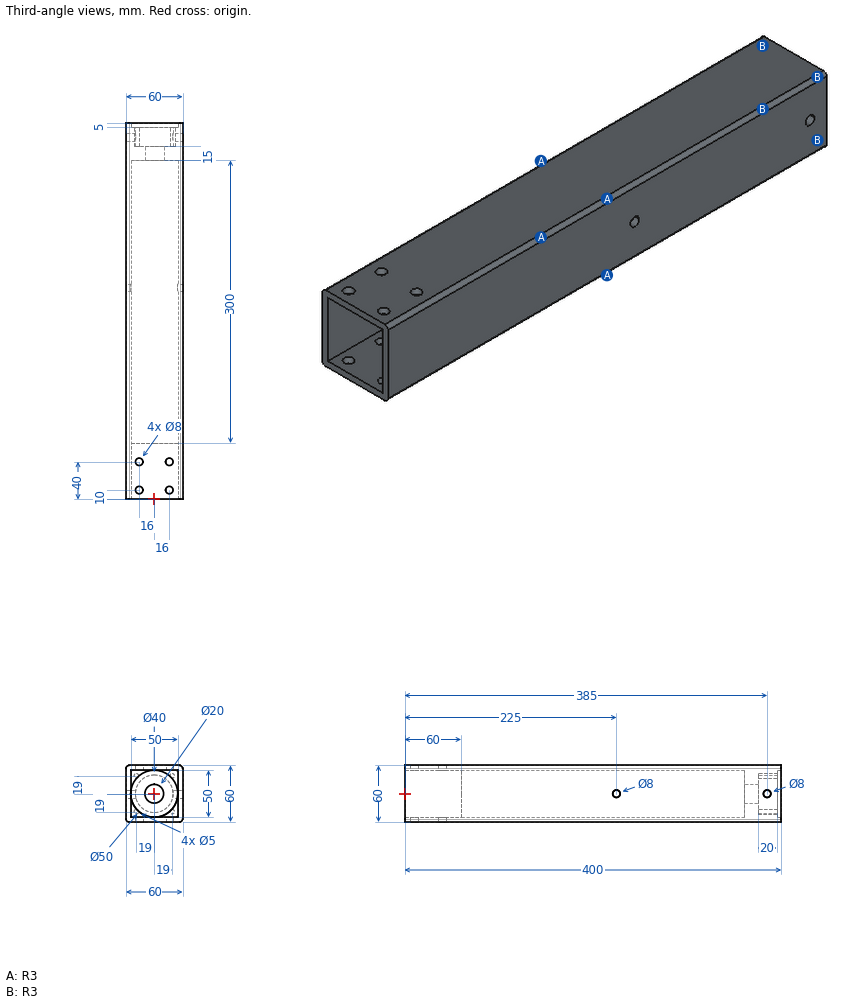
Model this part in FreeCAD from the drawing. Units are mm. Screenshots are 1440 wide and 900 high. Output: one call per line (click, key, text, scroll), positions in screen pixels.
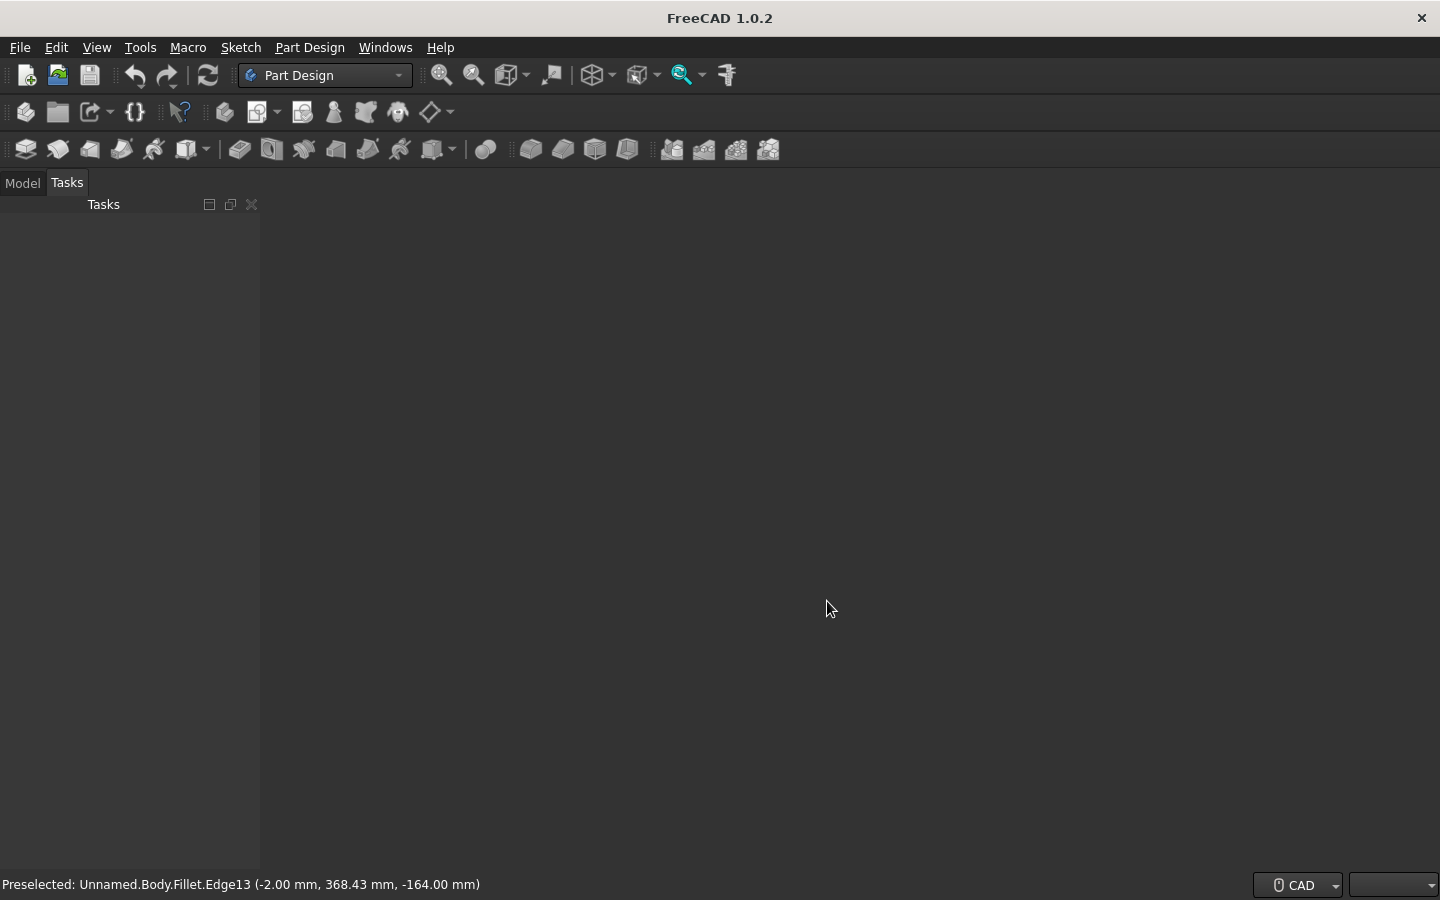
click(26, 76)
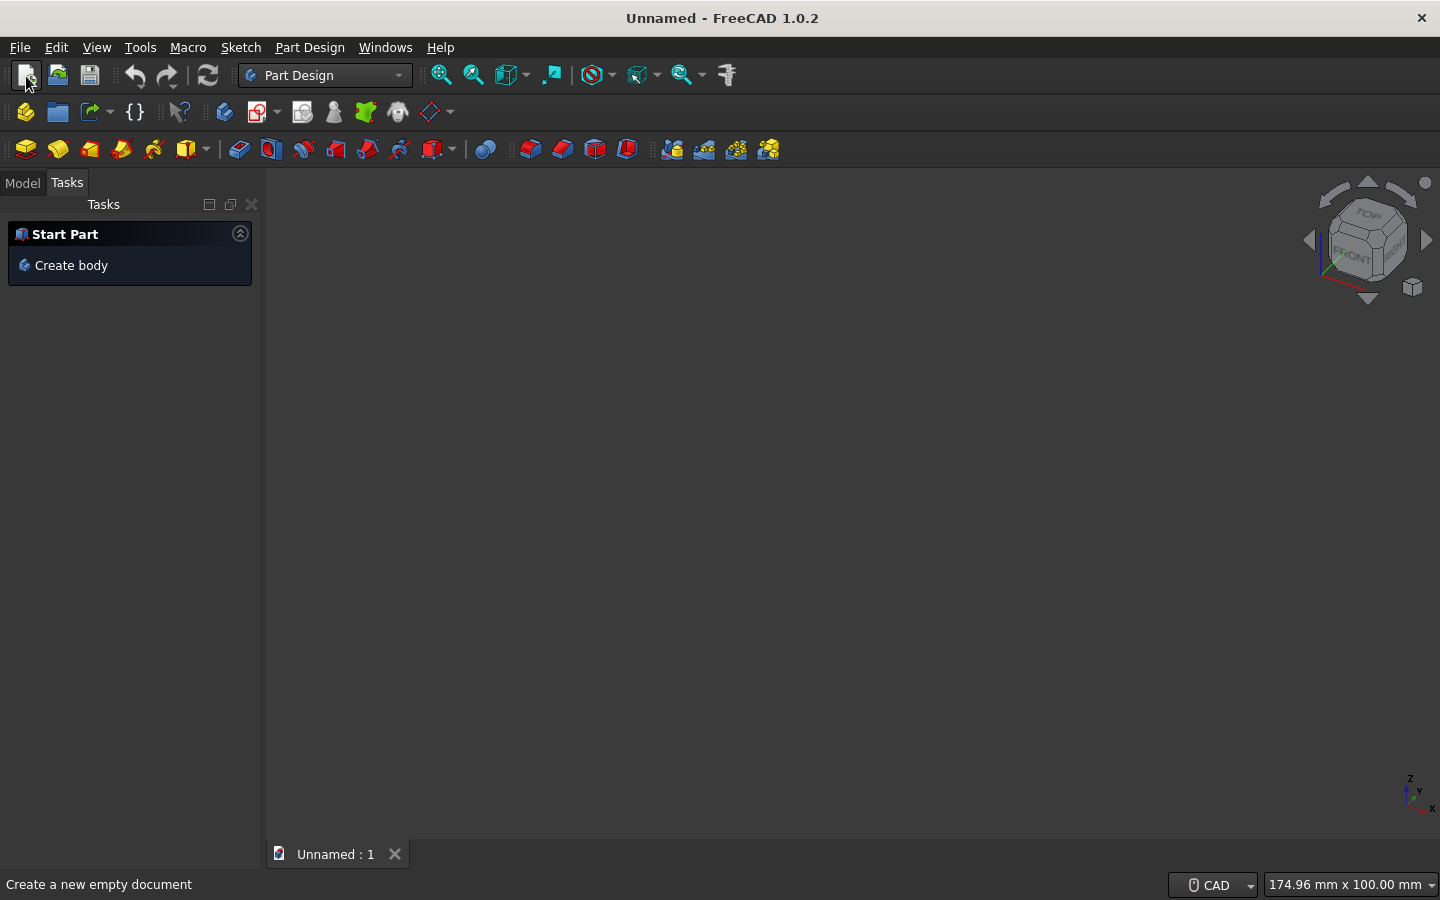
click(258, 112)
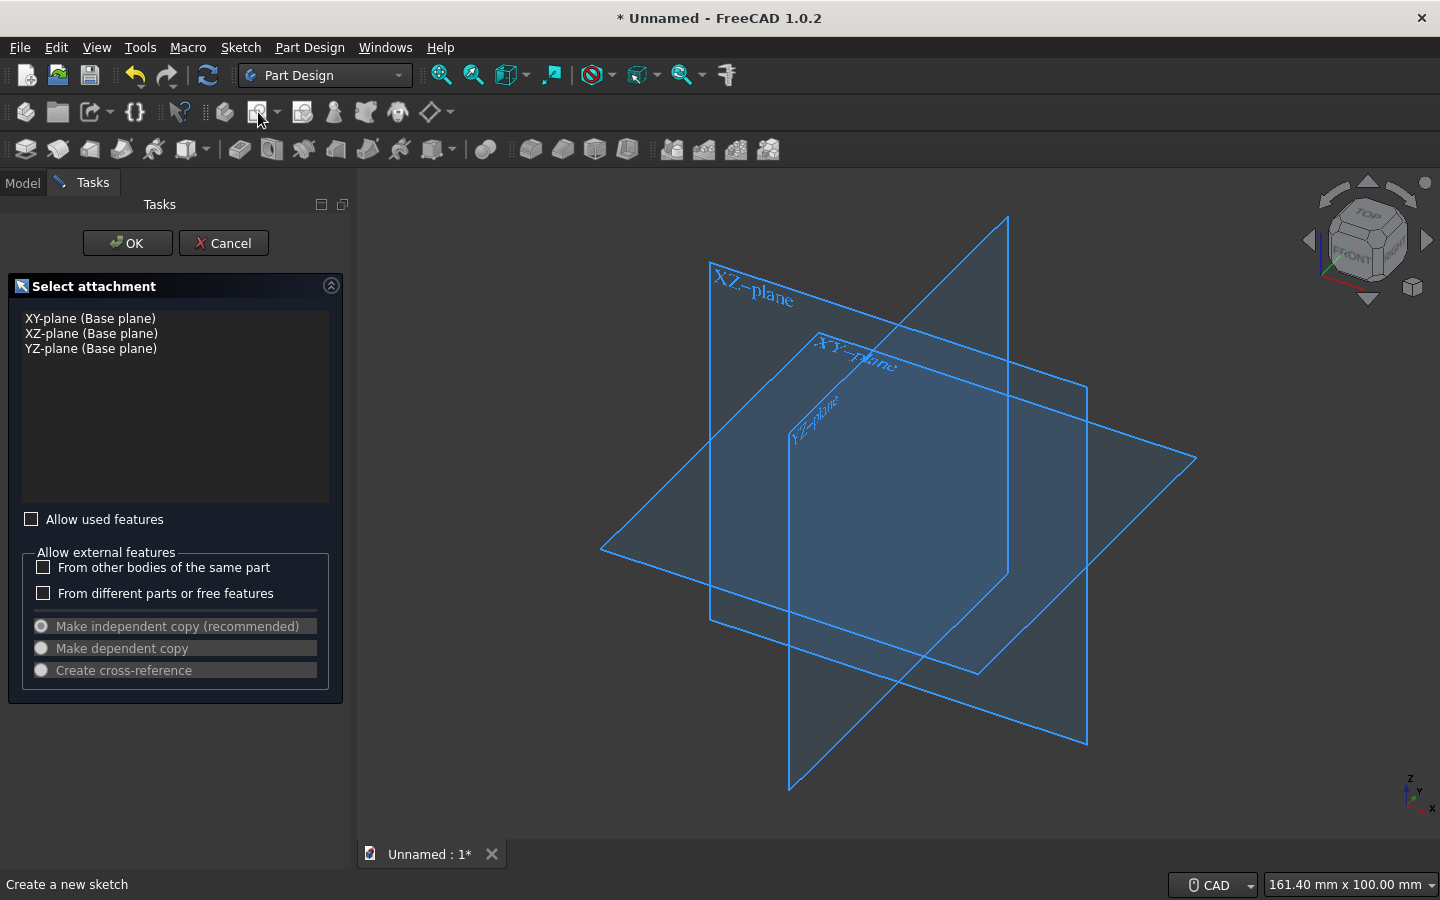
click(82, 334)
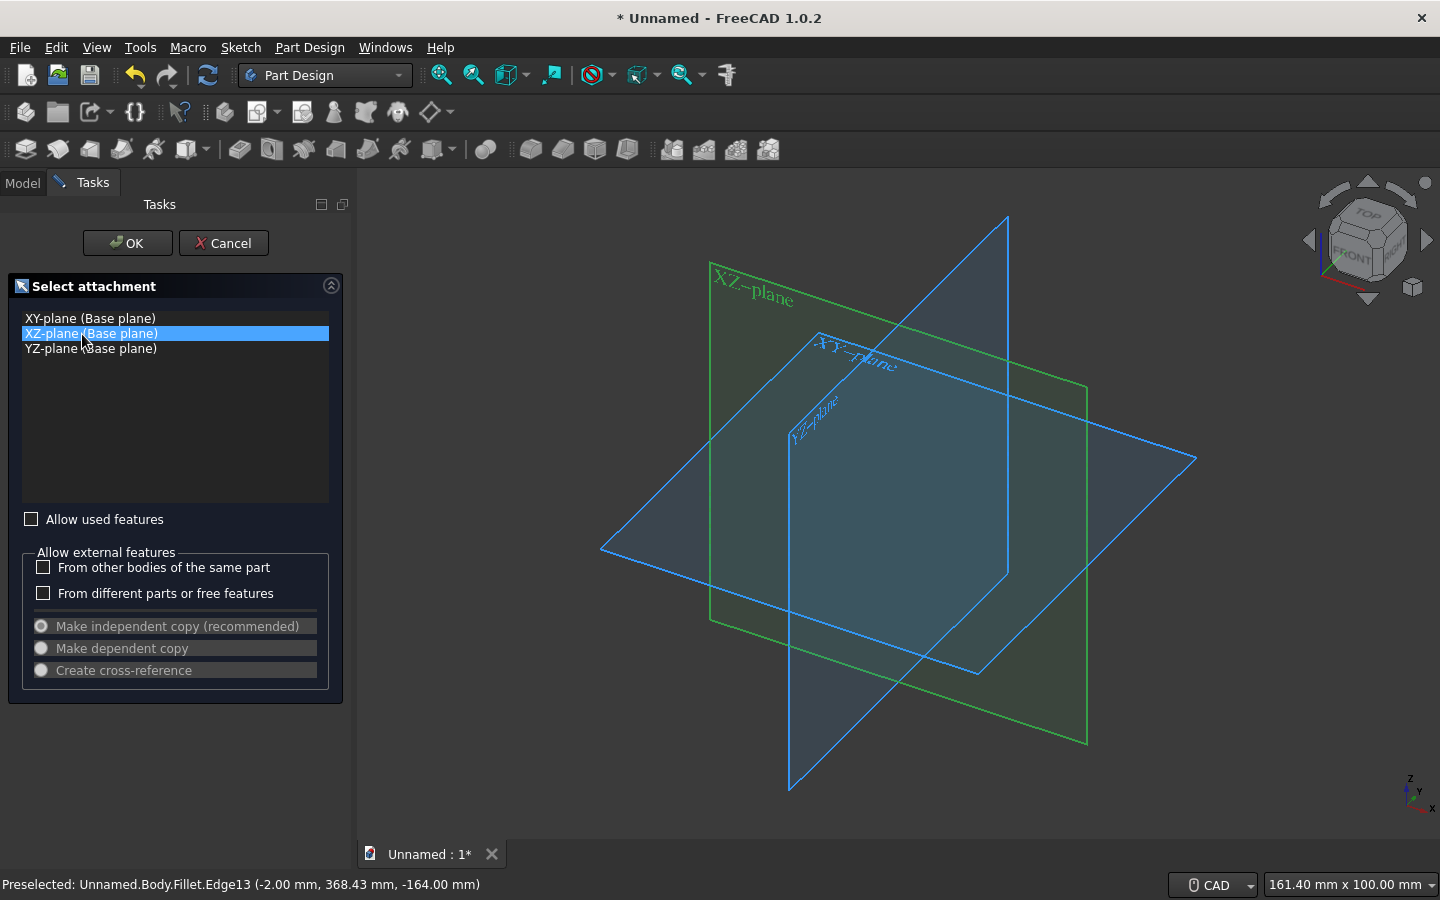
click(128, 243)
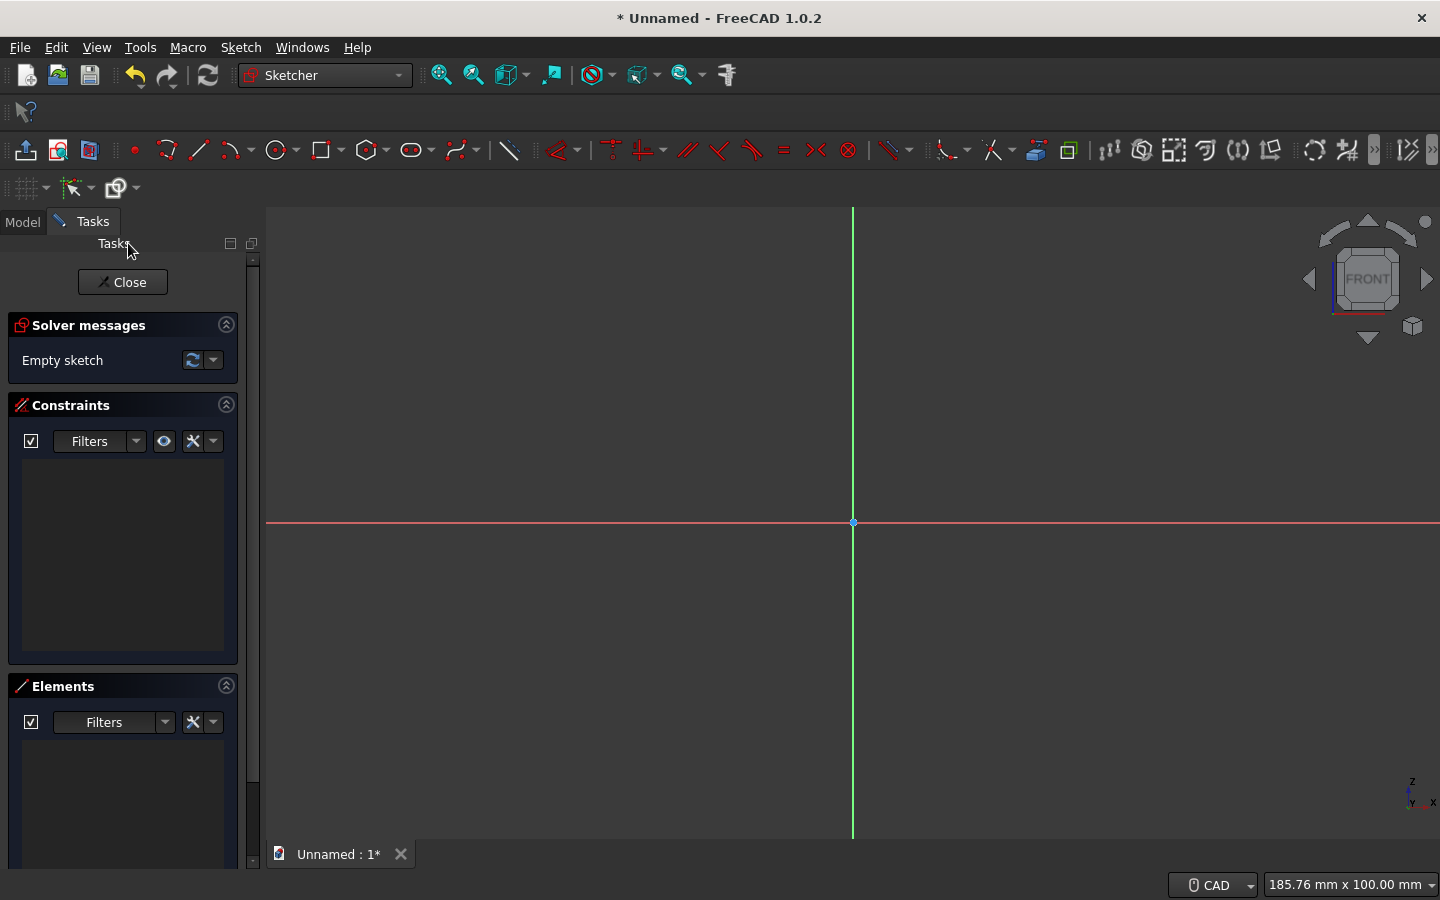
key(g)
key(v)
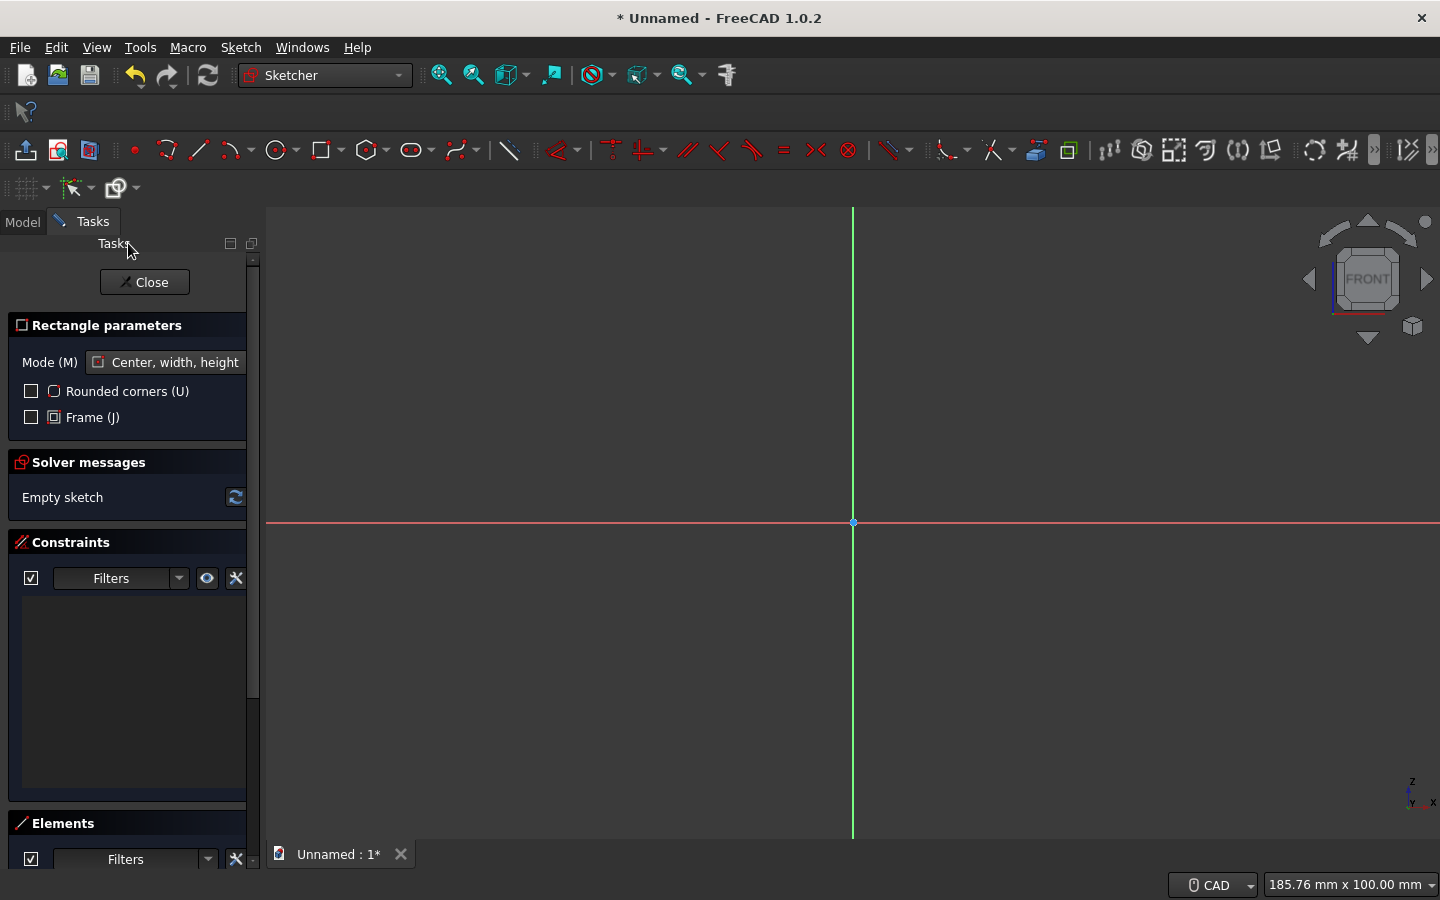
click(853, 523)
move(1043, 333)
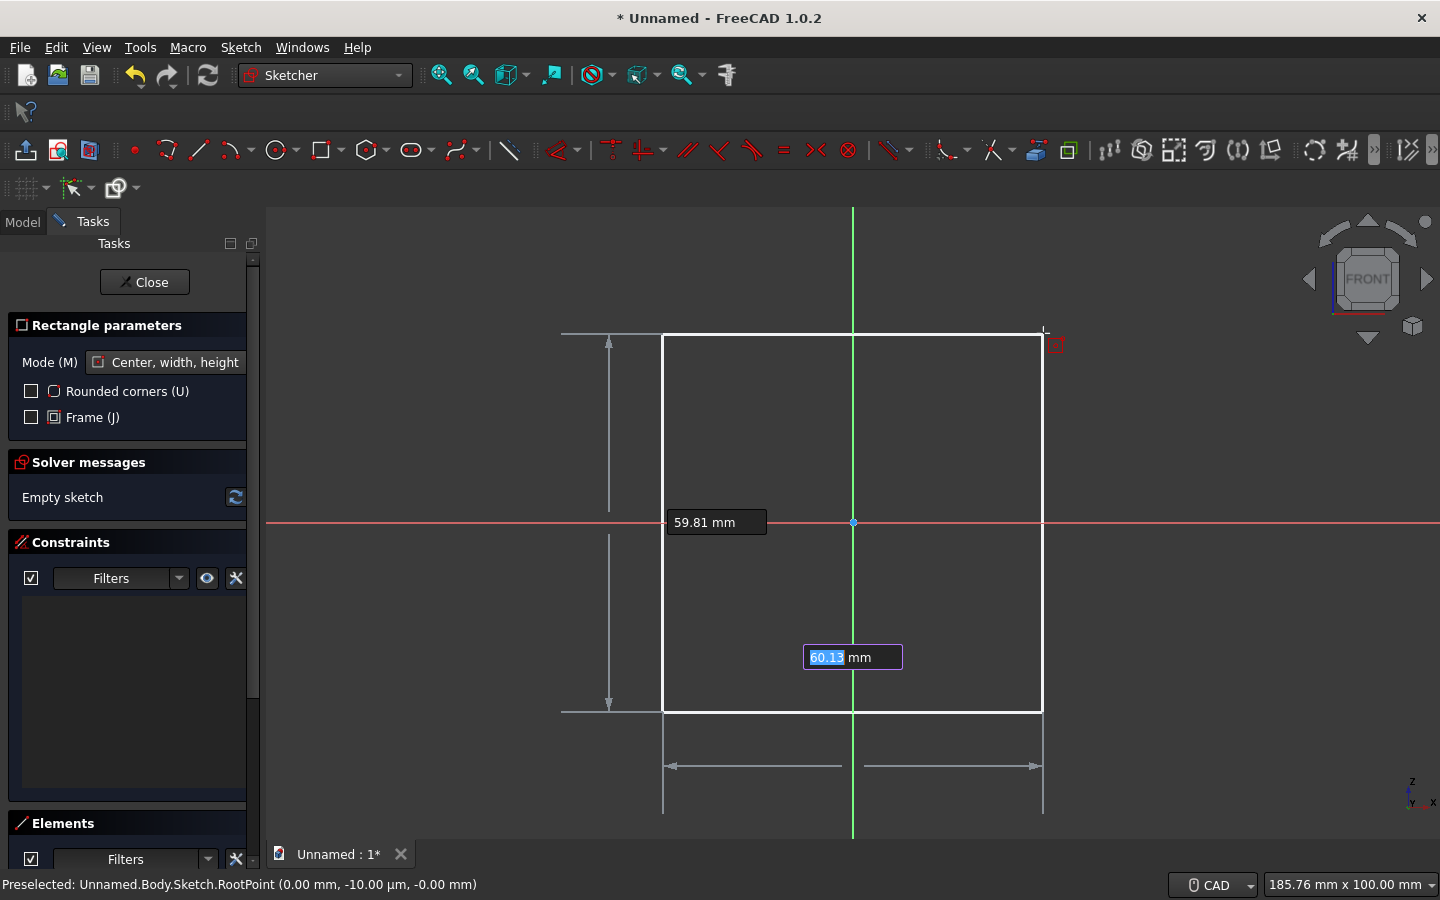
text(60)
key(Tab)
text(60)
key(Return)
key(Escape)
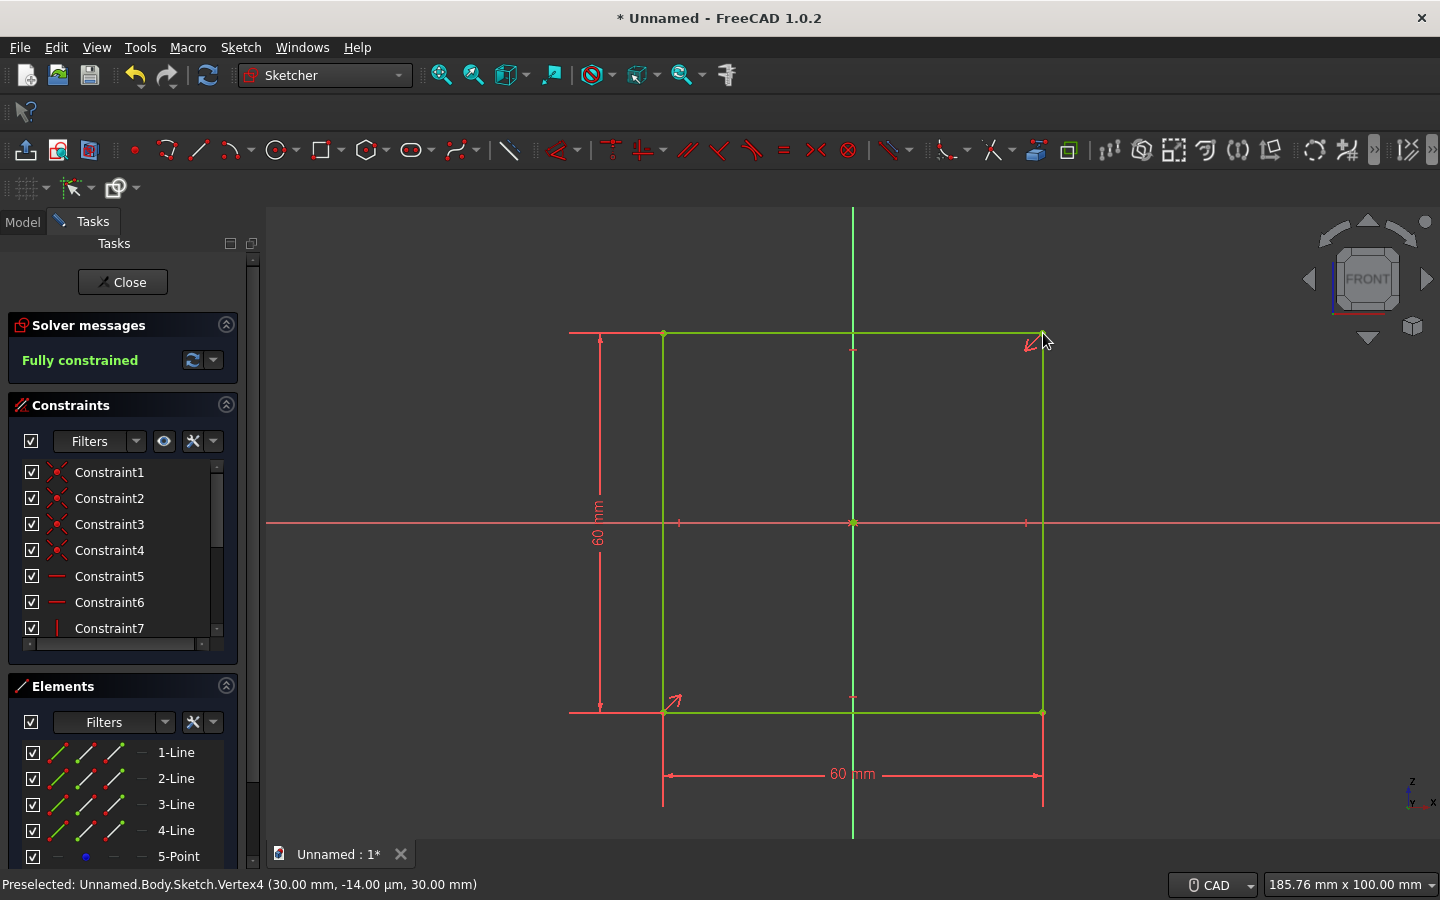
click(123, 282)